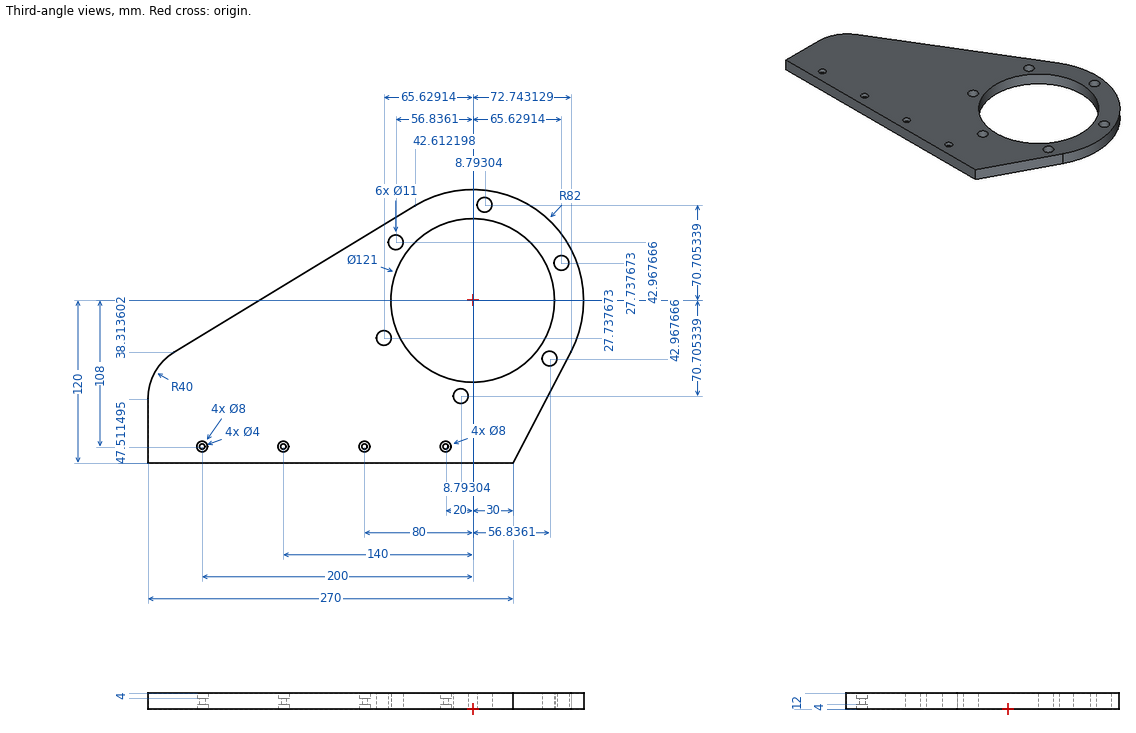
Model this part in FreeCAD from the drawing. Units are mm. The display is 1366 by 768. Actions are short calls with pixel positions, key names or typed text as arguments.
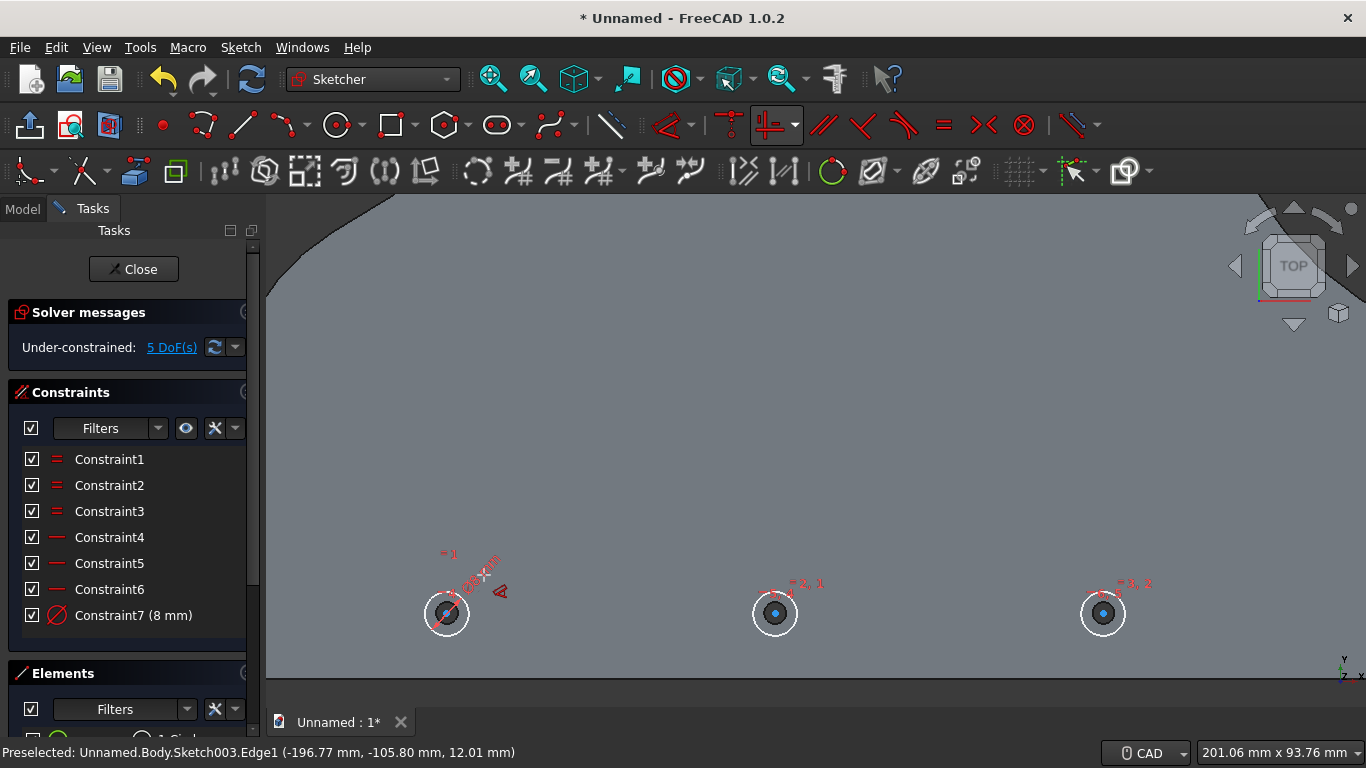
click(1103, 614)
click(1152, 648)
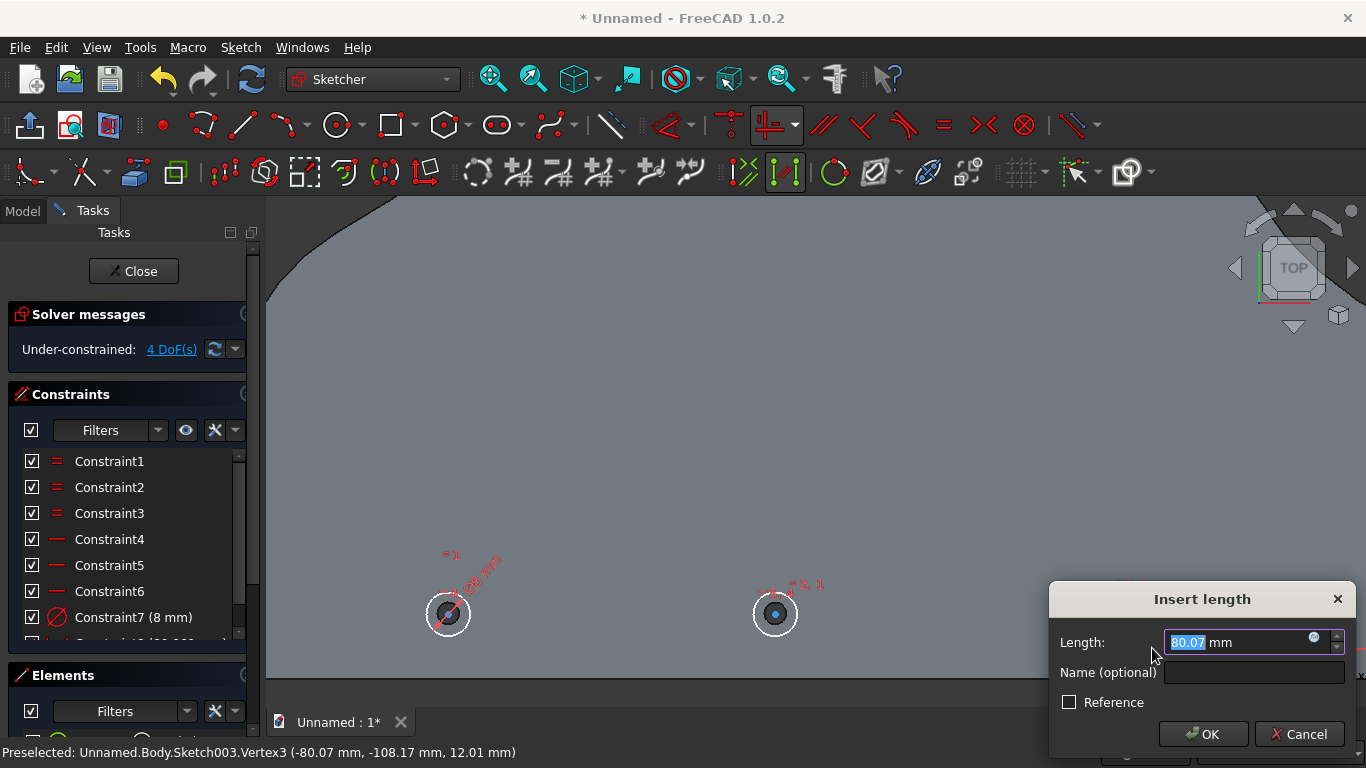
text(80)
key(Return)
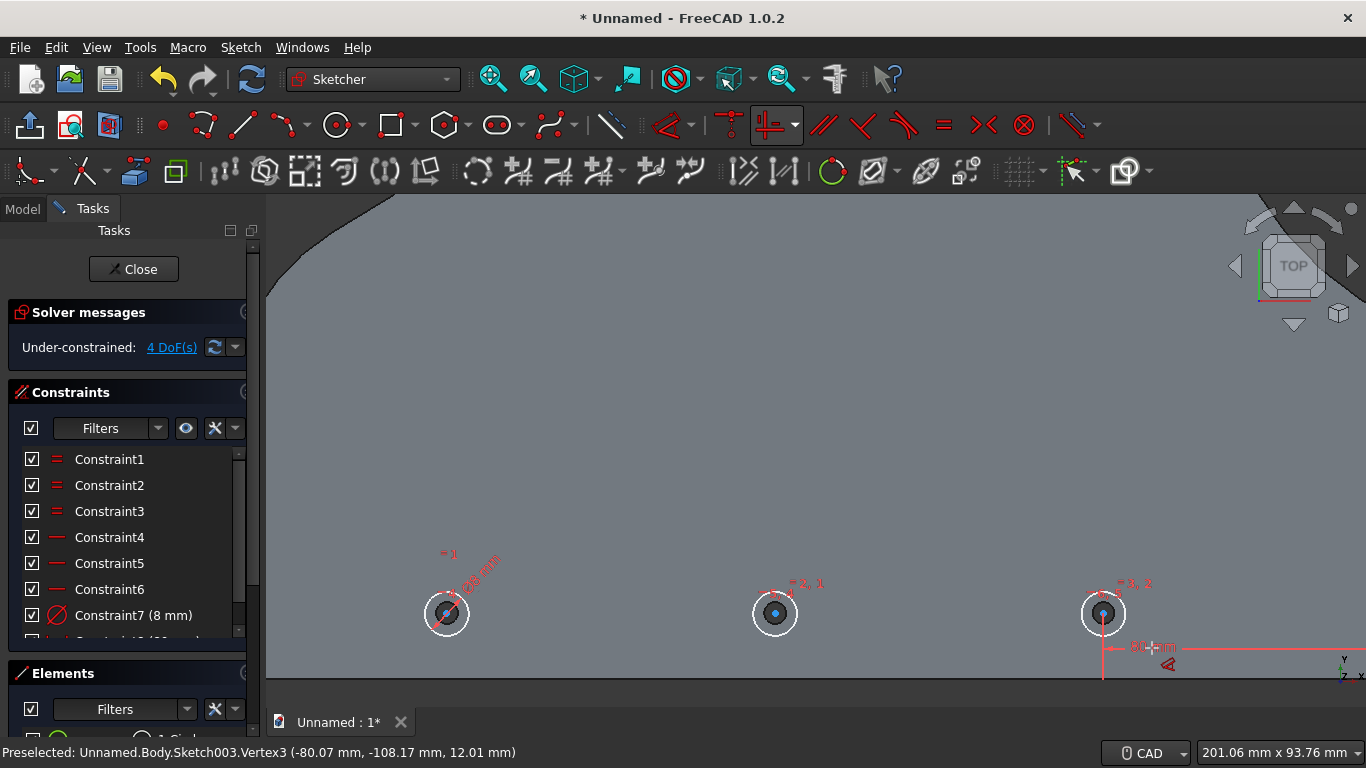
scroll(461, 599, down, 3)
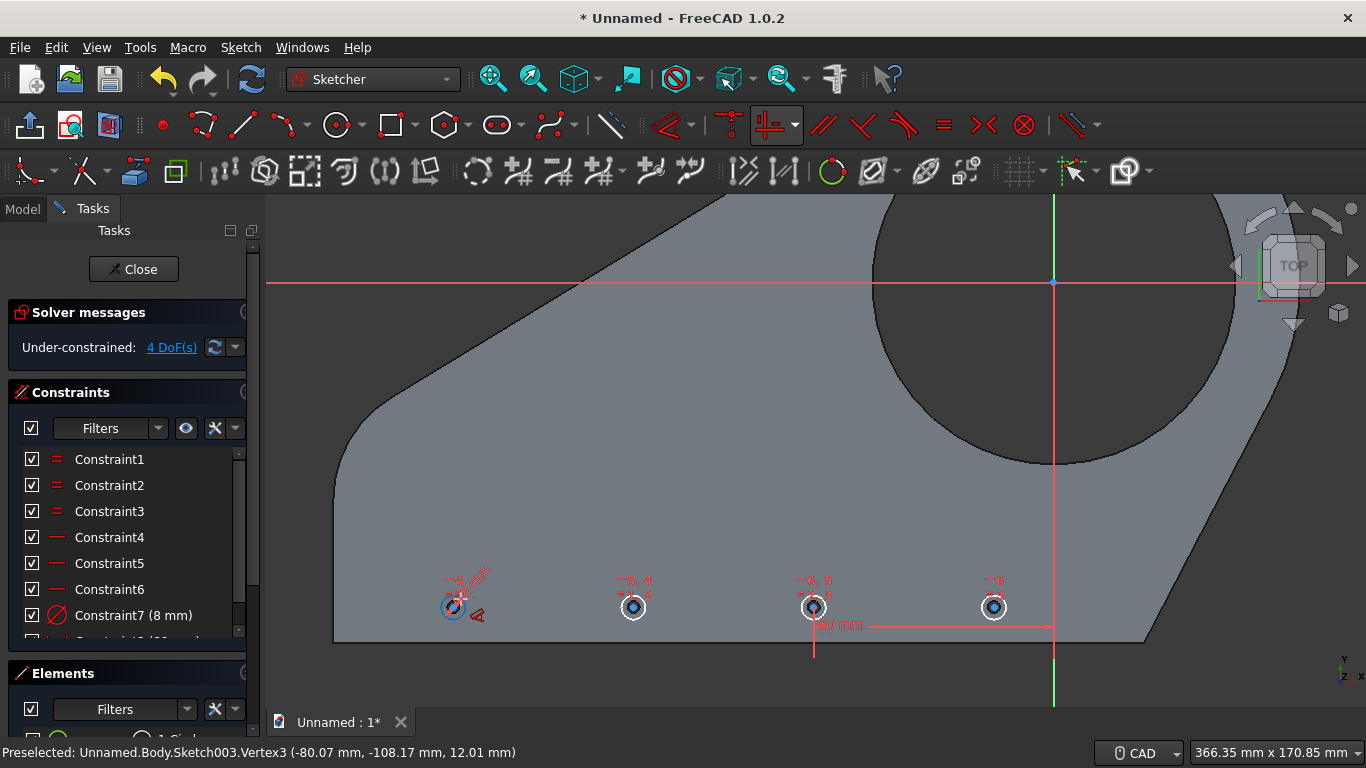
click(994, 608)
click(1024, 249)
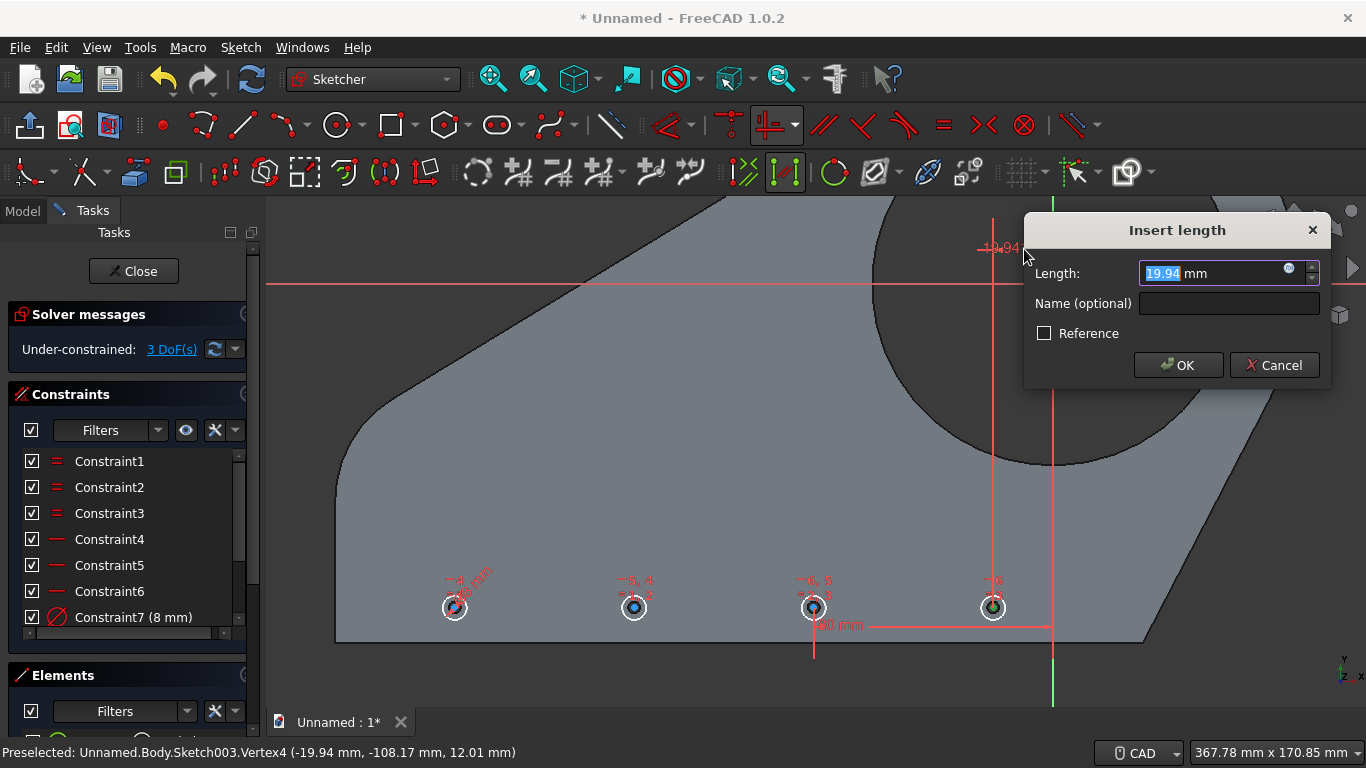
text(20)
key(Return)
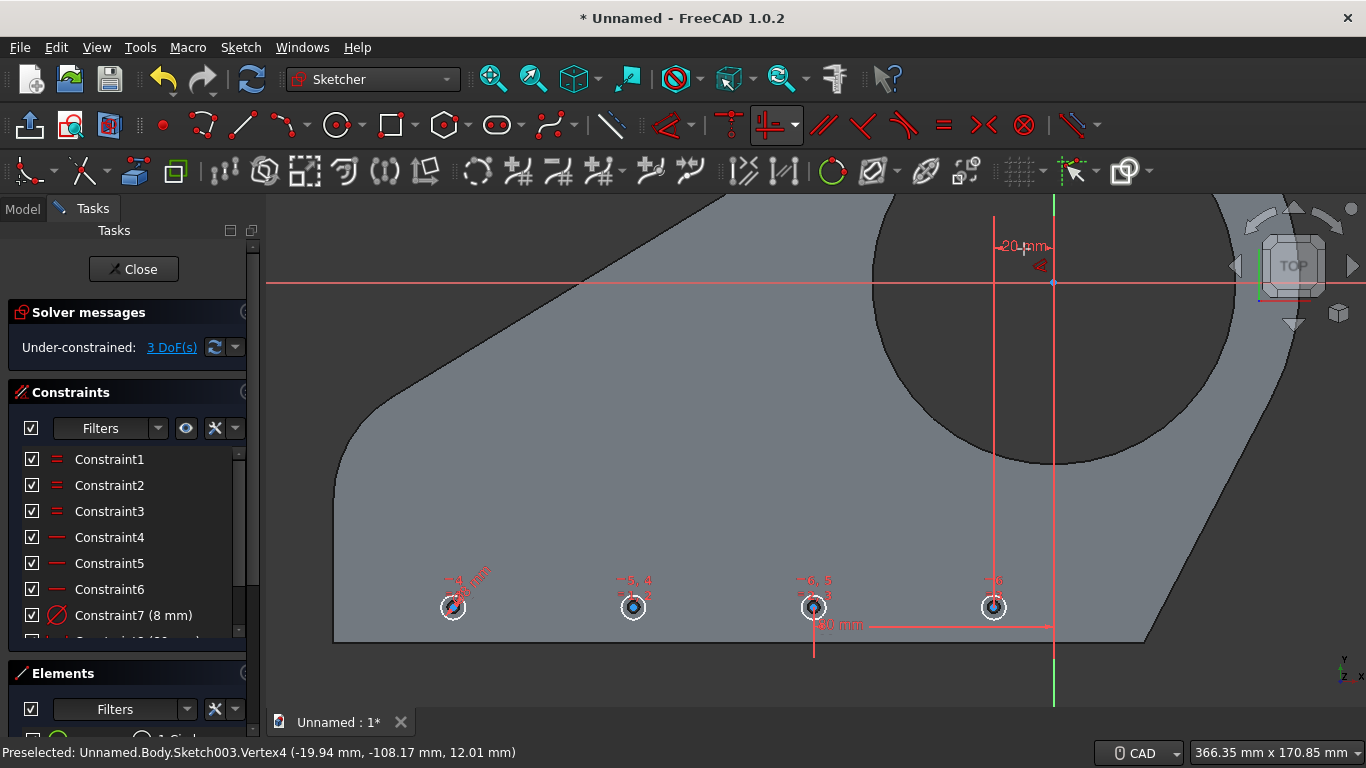
click(453, 608)
click(754, 249)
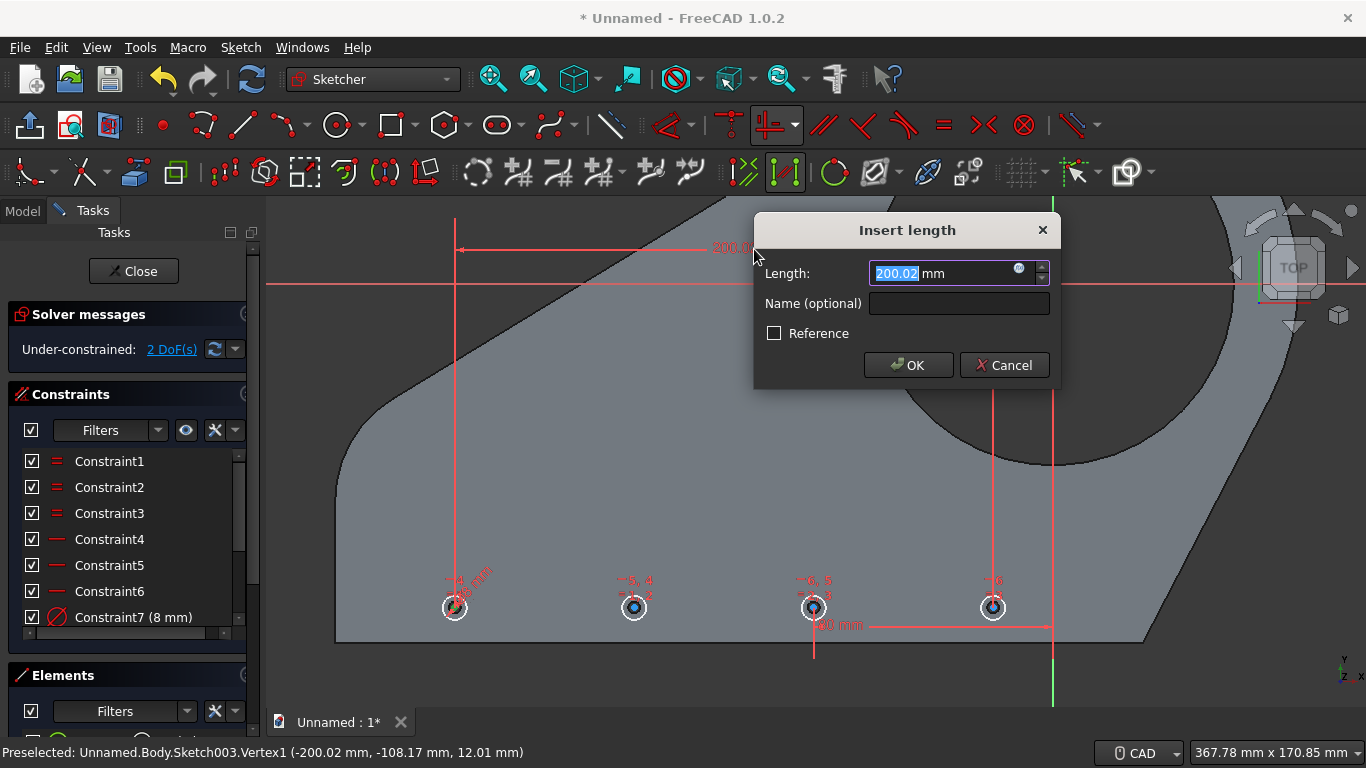
text(200)
key(Return)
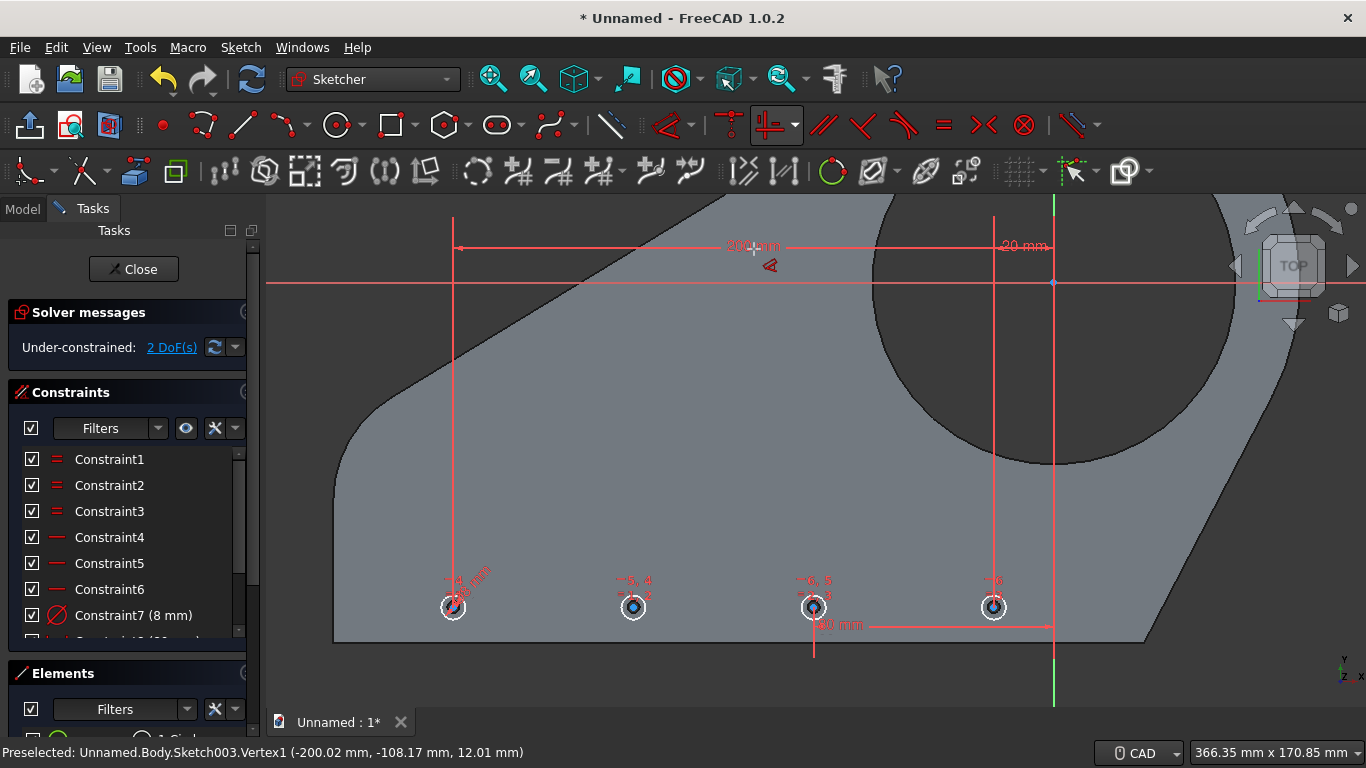
click(453, 608)
click(1088, 445)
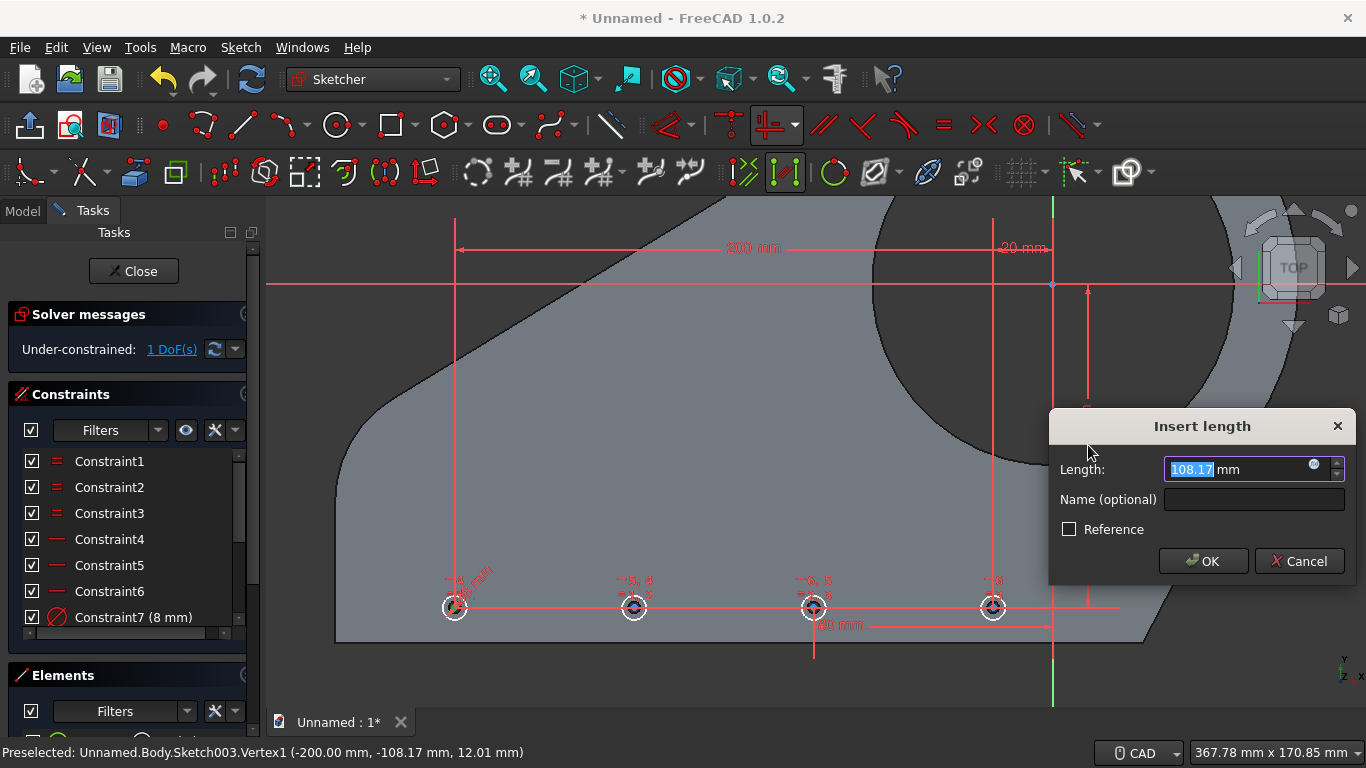
text(108)
key(Return)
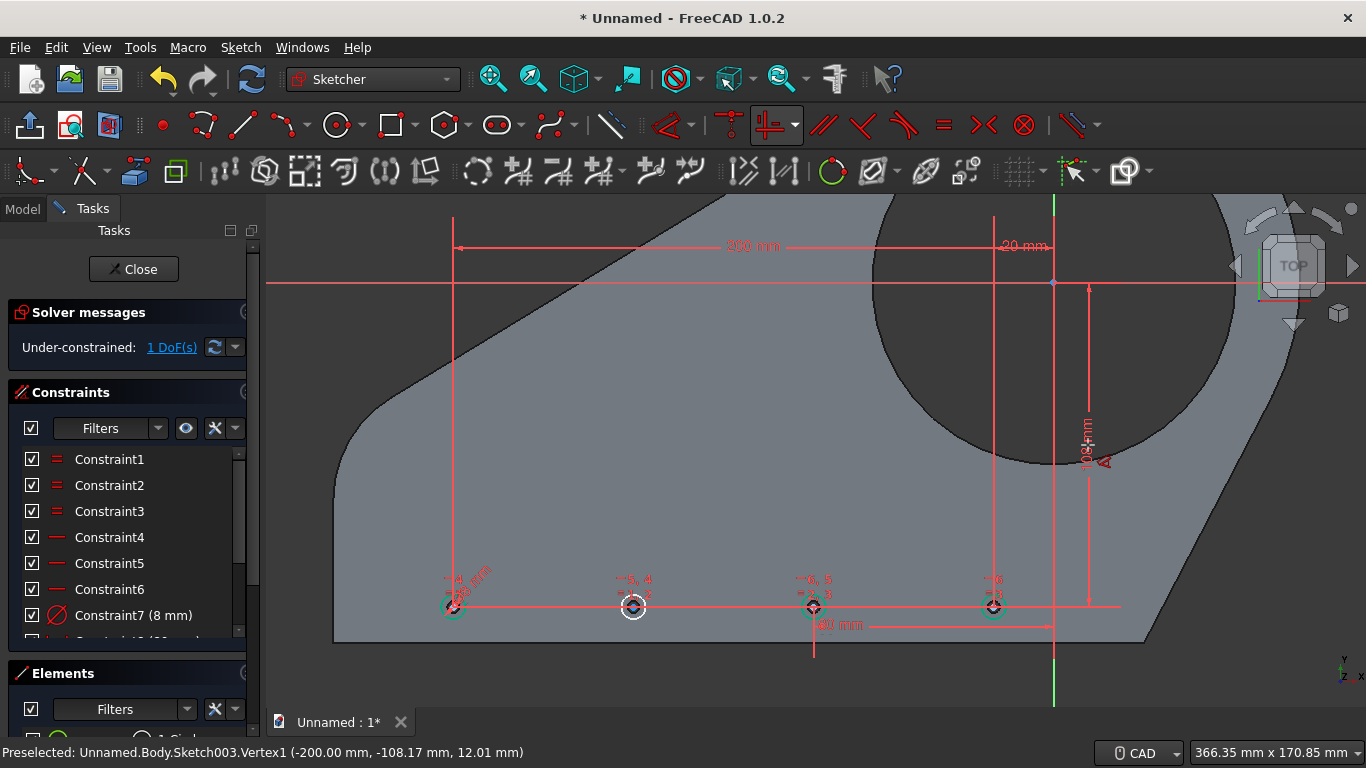
click(633, 607)
click(844, 249)